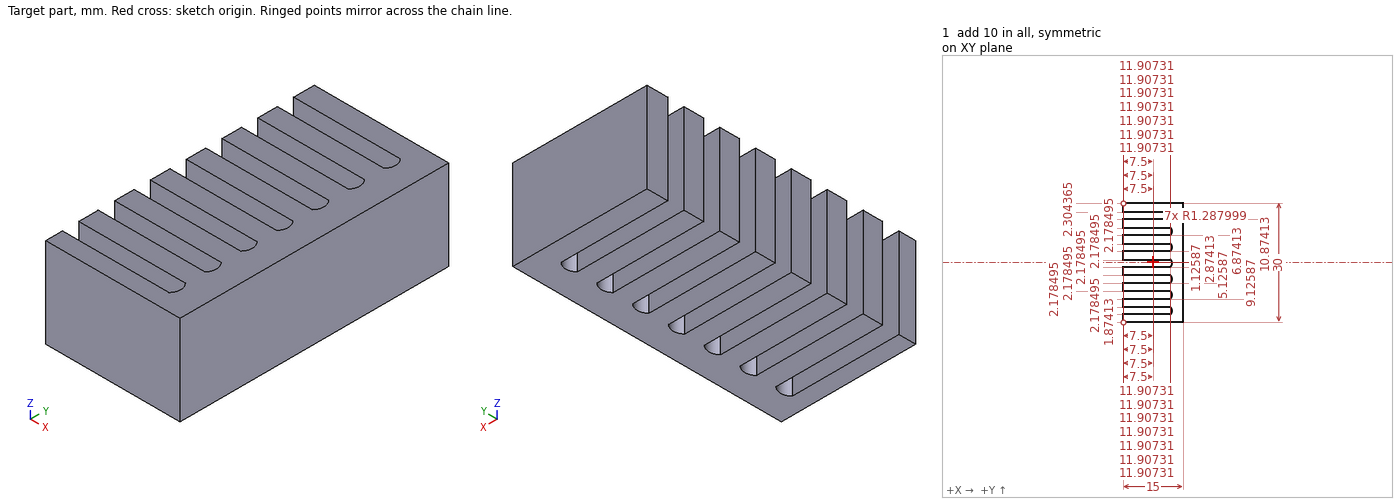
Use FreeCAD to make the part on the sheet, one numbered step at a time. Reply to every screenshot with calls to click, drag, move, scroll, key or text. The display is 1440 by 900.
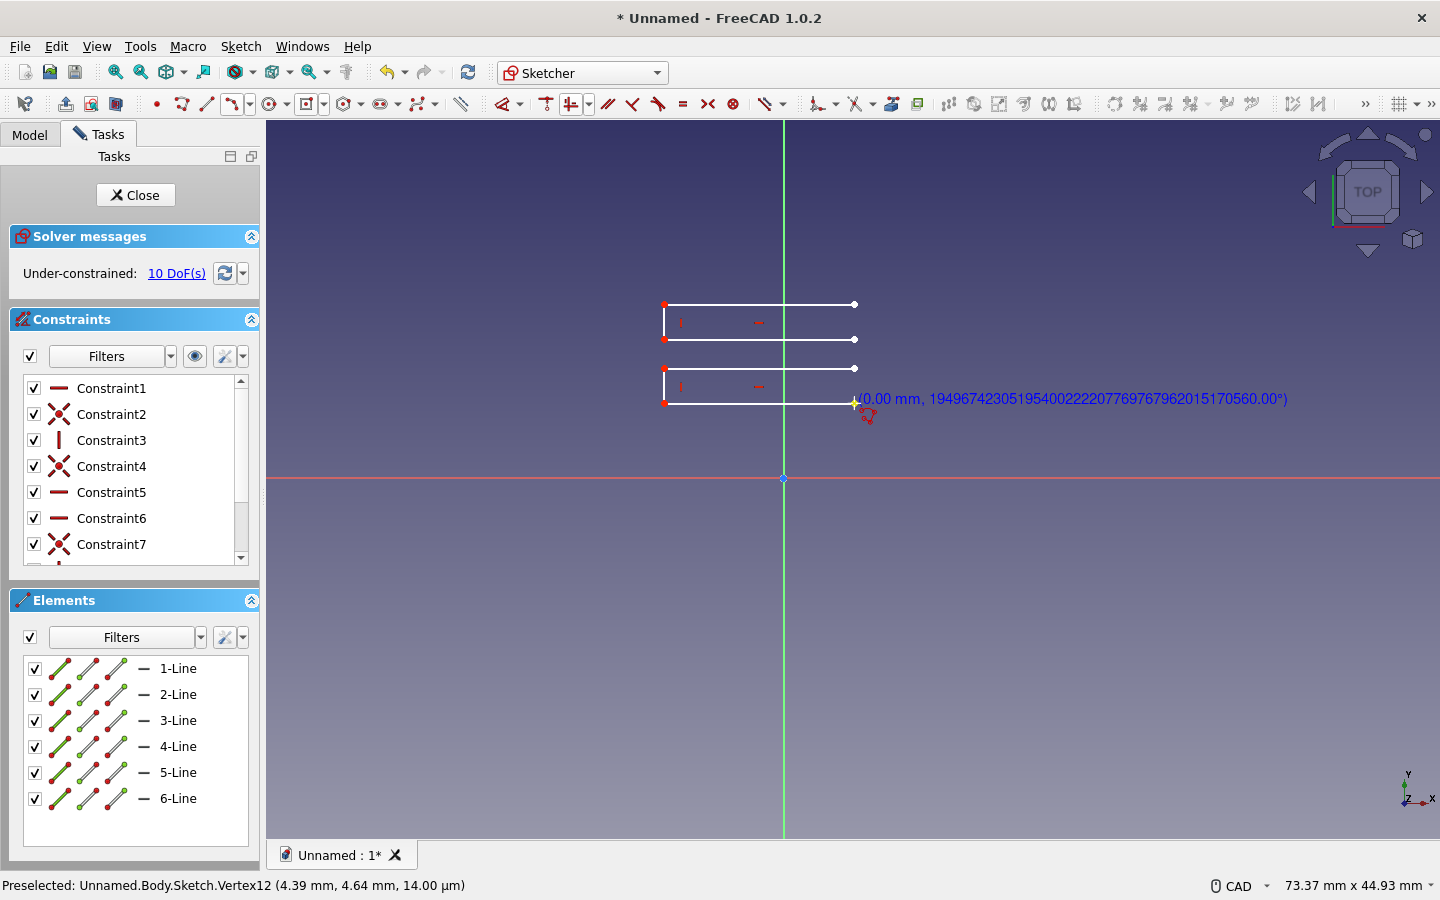
click(854, 432)
click(664, 432)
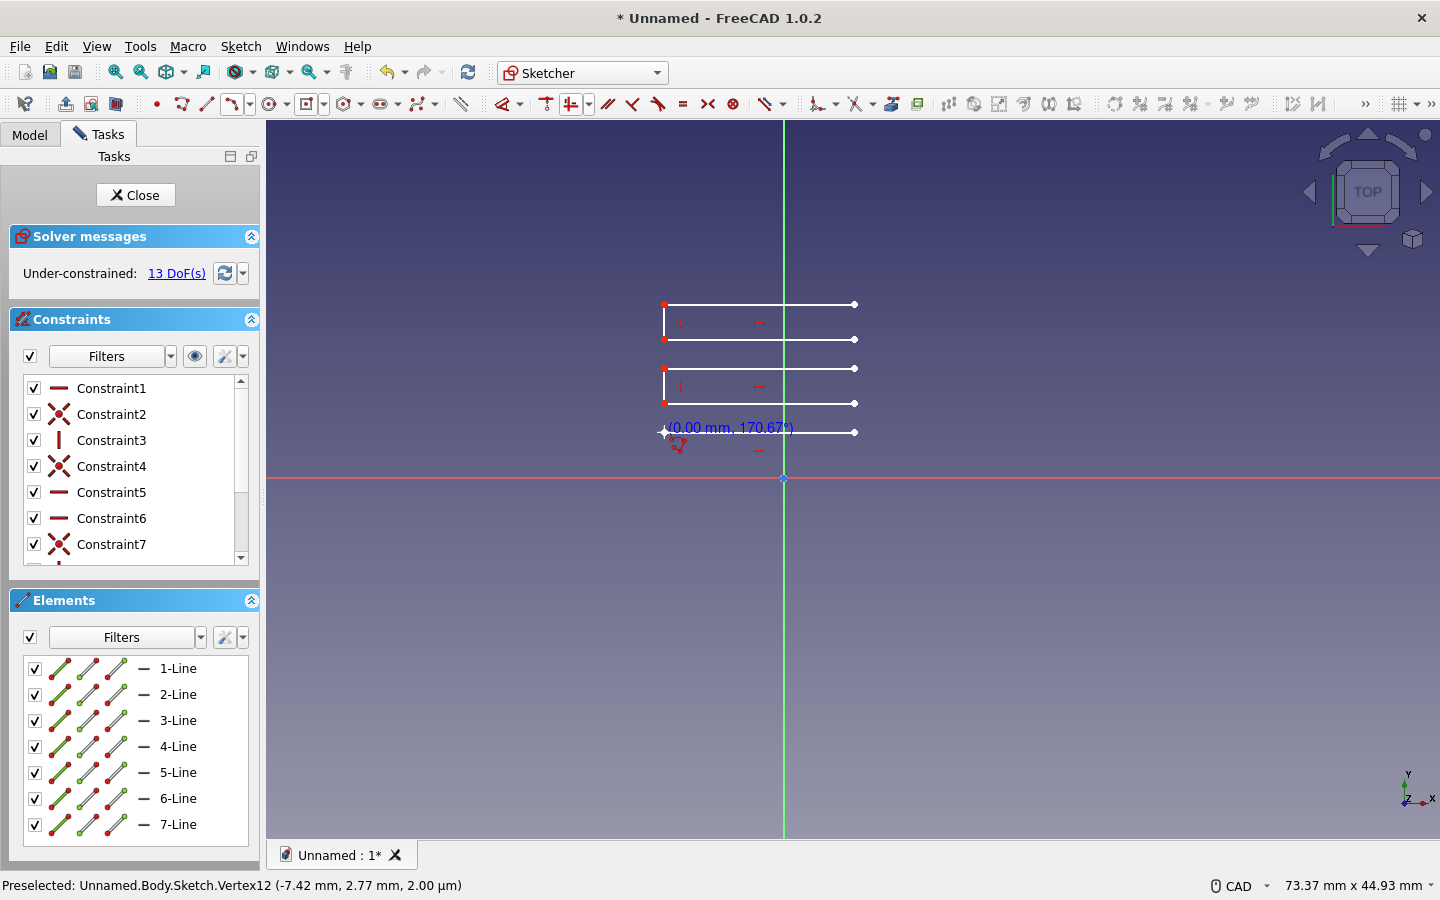
scroll(664, 467, up, 2)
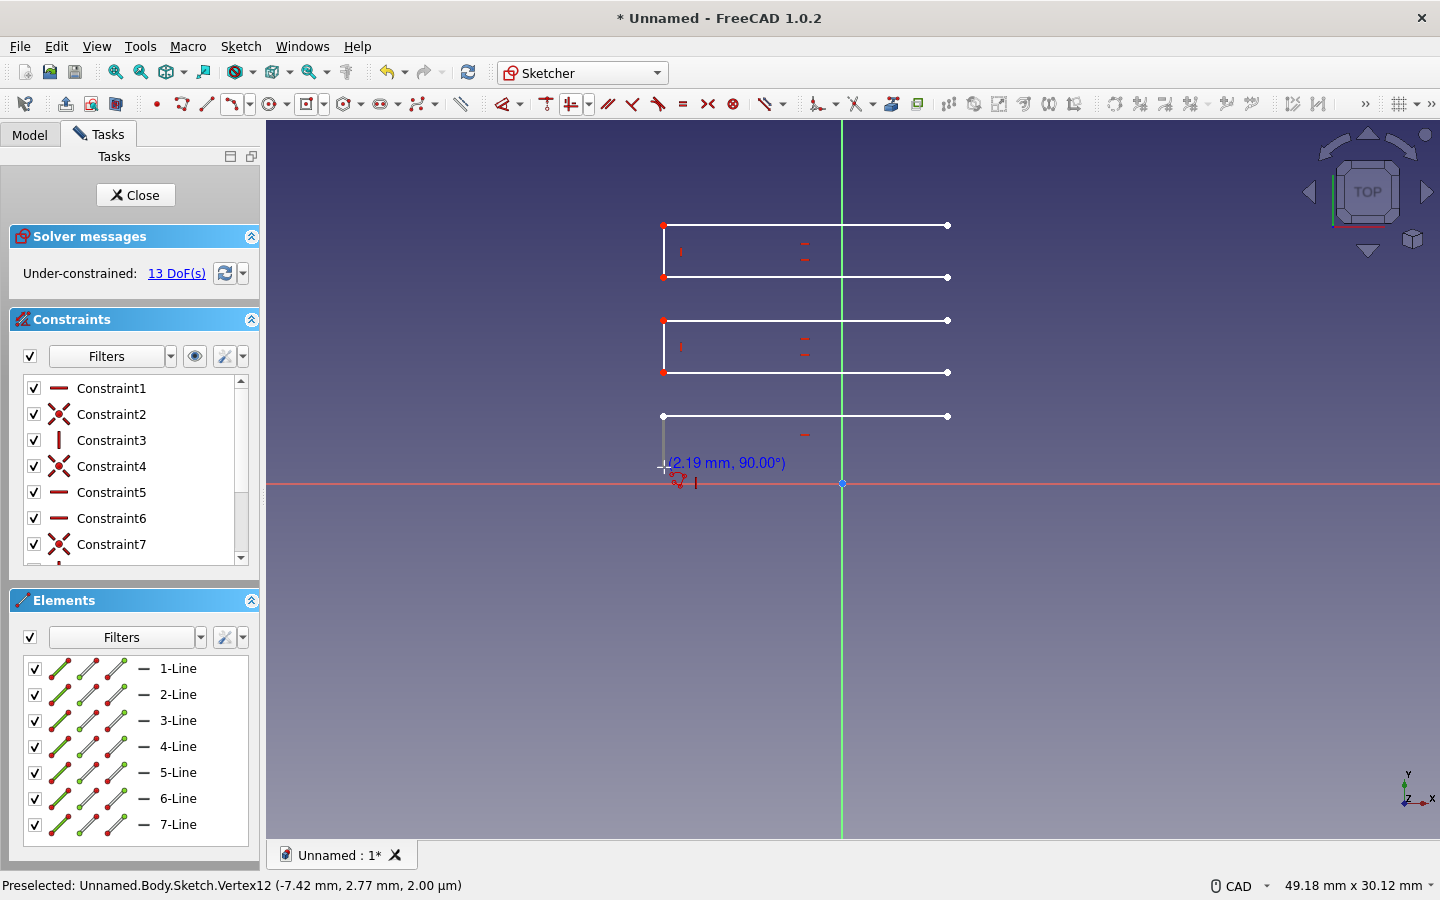
click(664, 467)
click(948, 467)
right_click(948, 467)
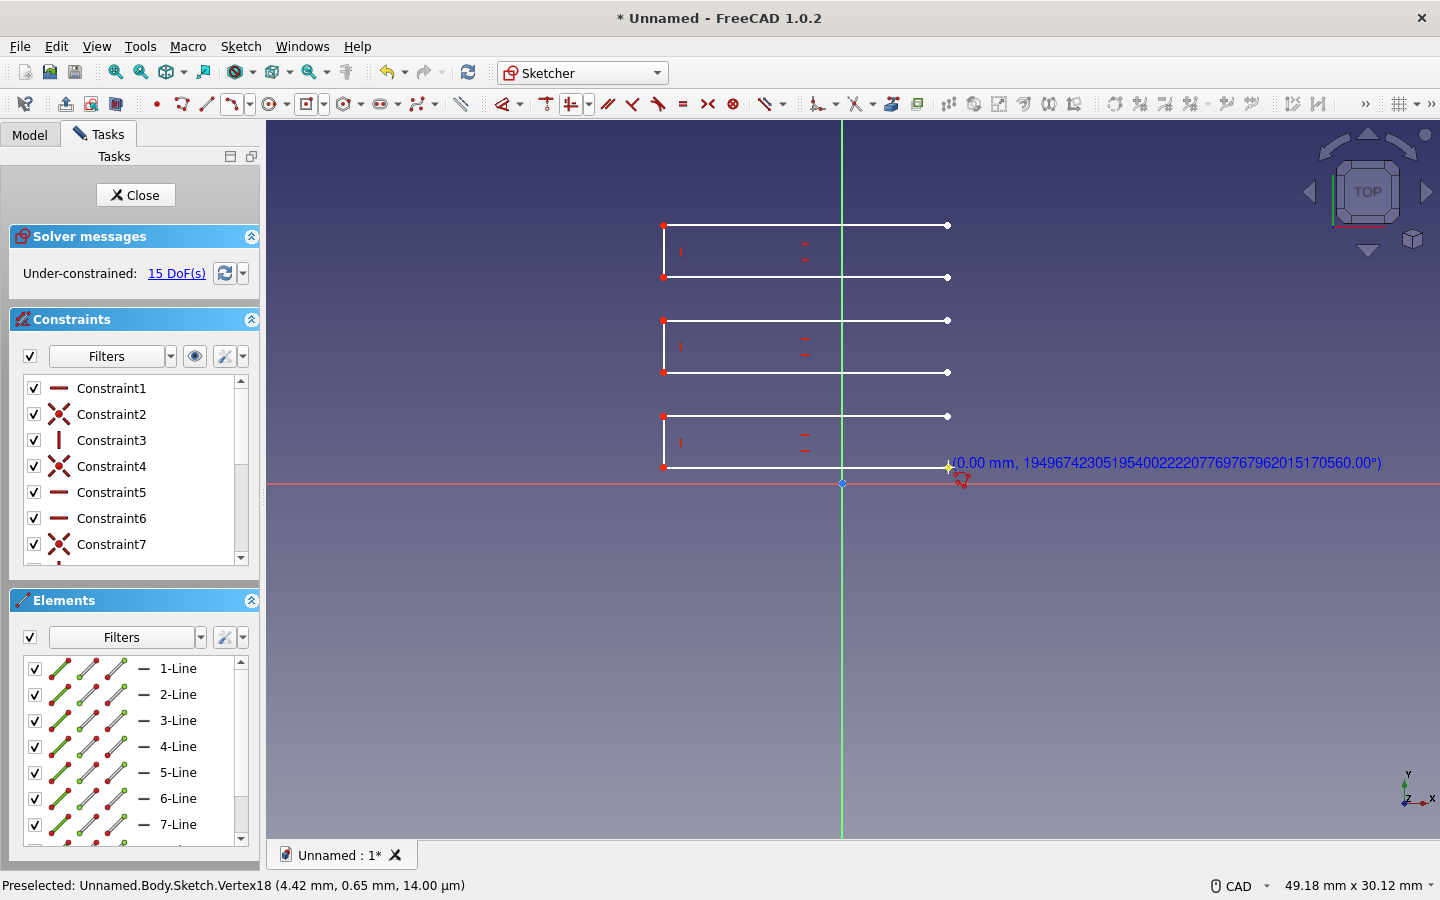
click(948, 510)
click(663, 510)
click(663, 562)
click(948, 562)
right_click(948, 562)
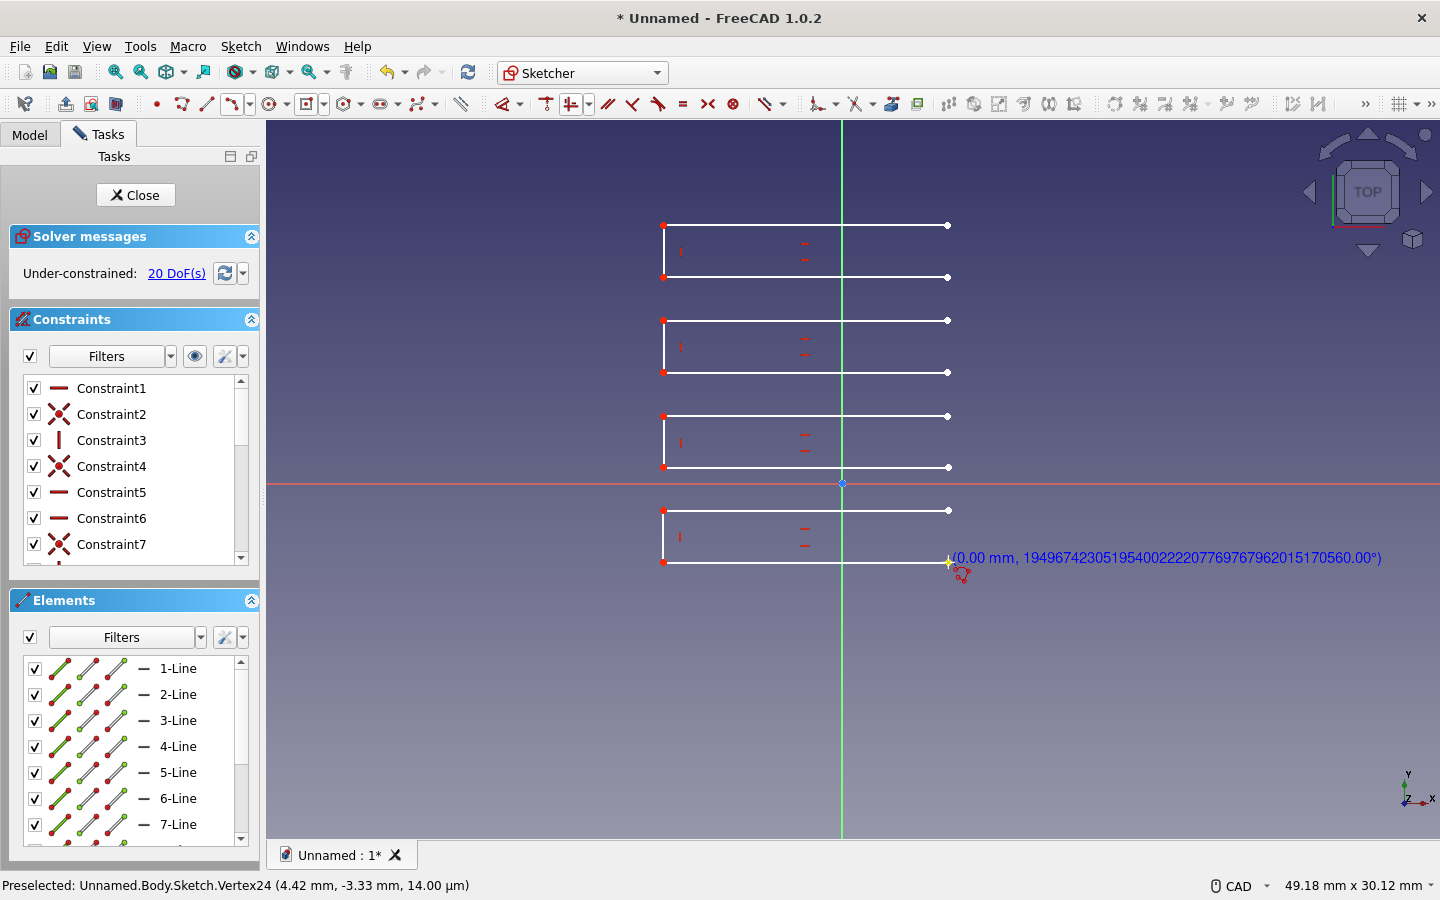
click(948, 606)
click(663, 606)
click(663, 658)
click(948, 658)
right_click(948, 658)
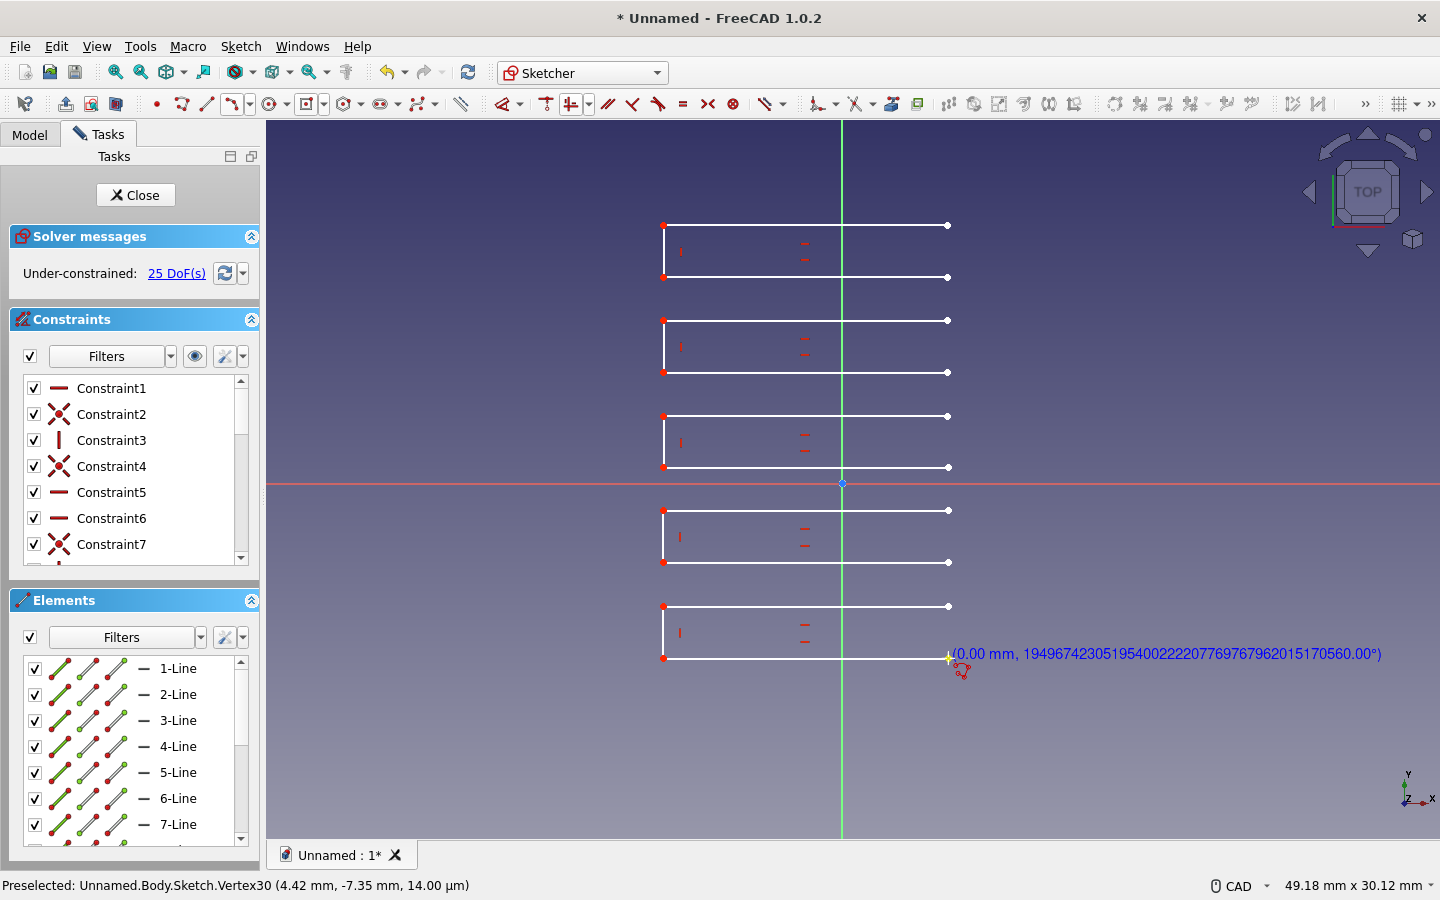
click(948, 701)
click(663, 701)
click(663, 753)
click(948, 753)
right_click(948, 753)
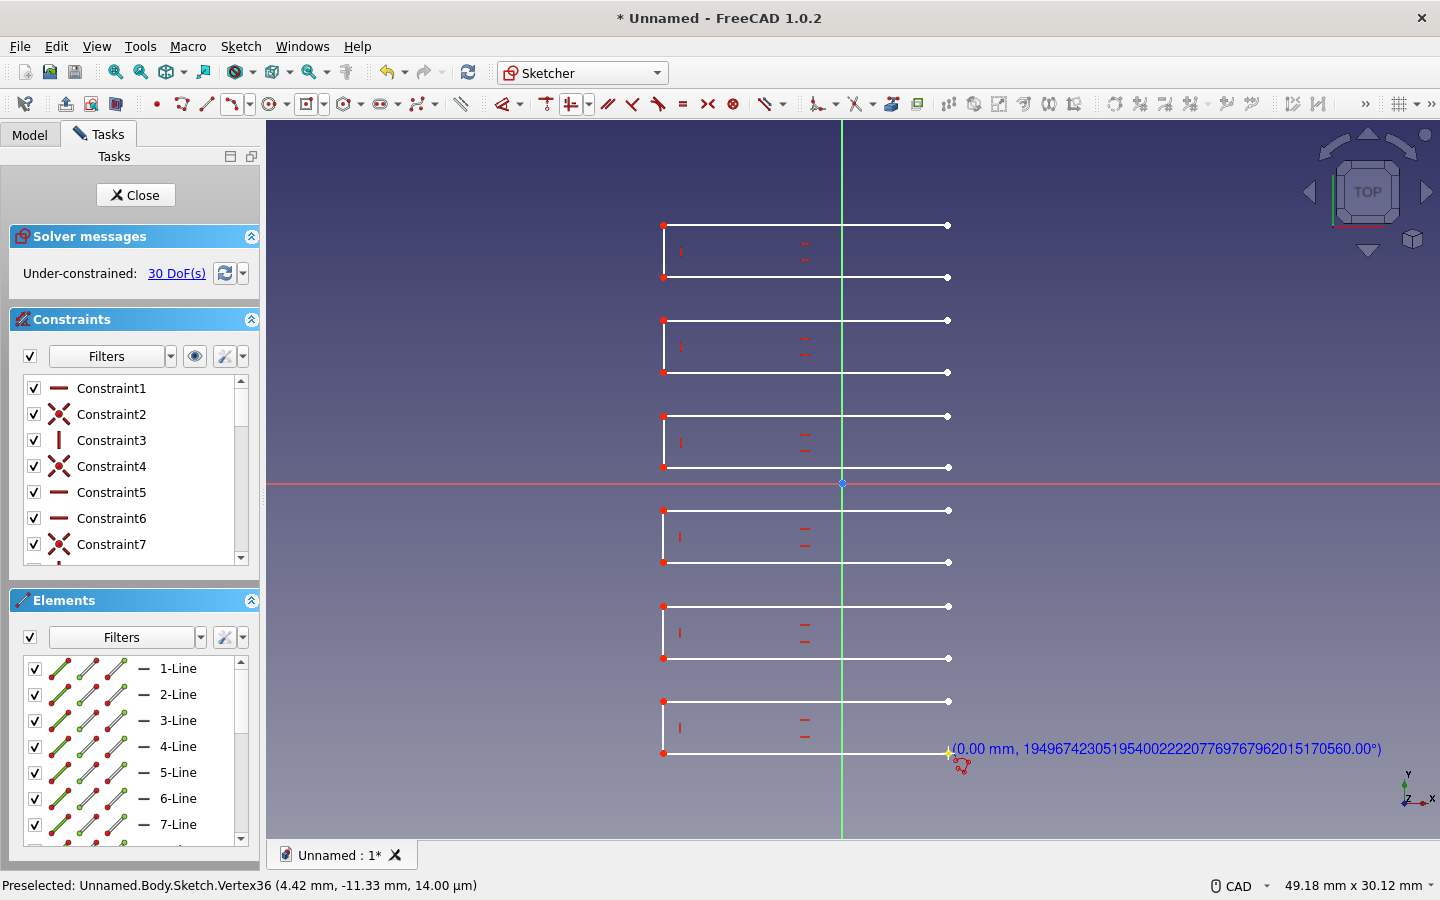
click(948, 797)
click(663, 797)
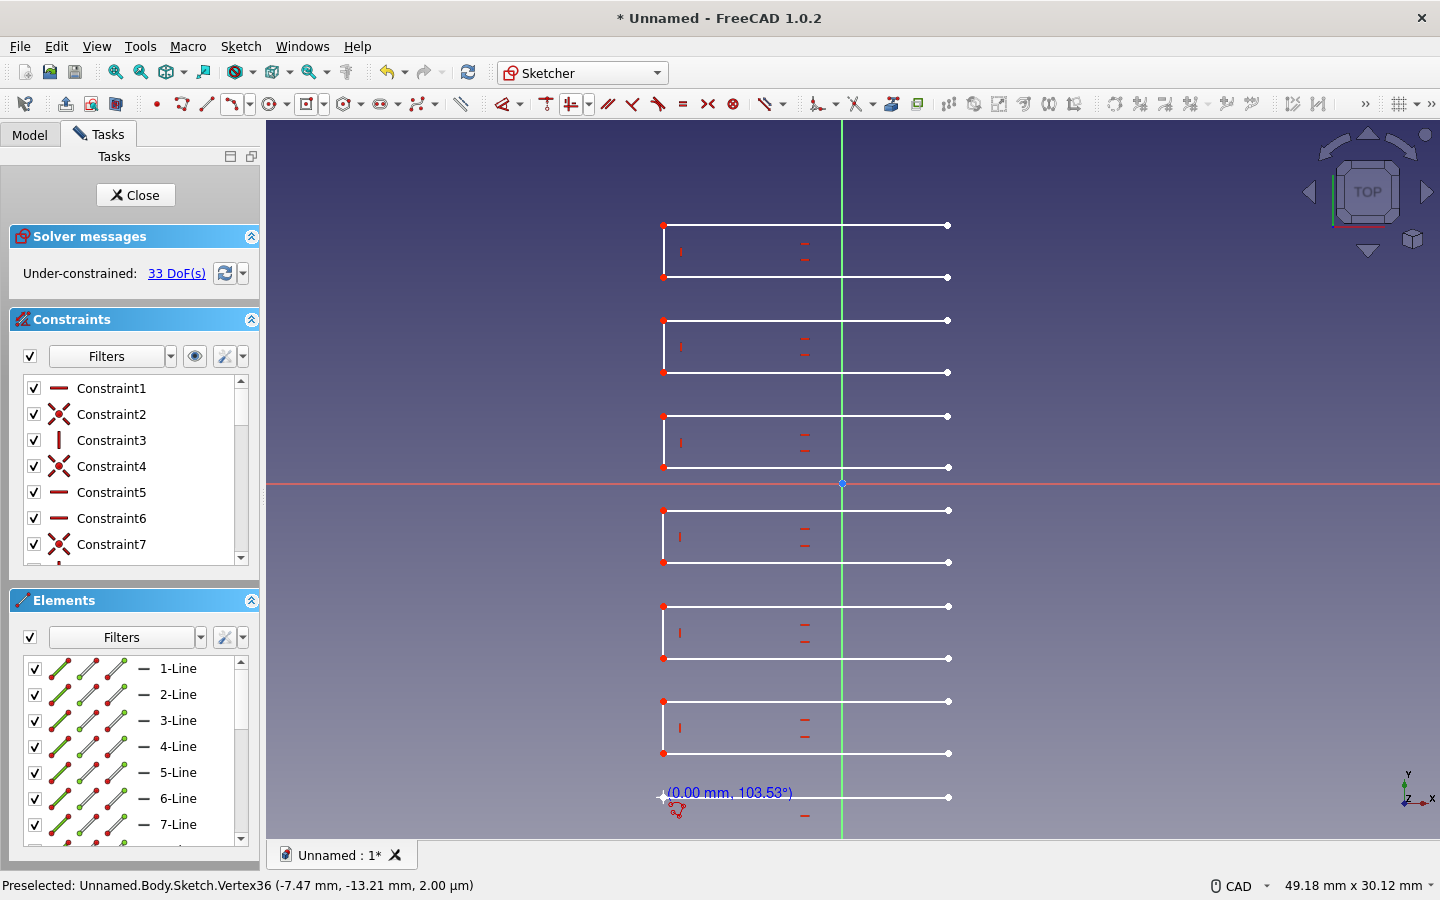
scroll(667, 471, down, 2)